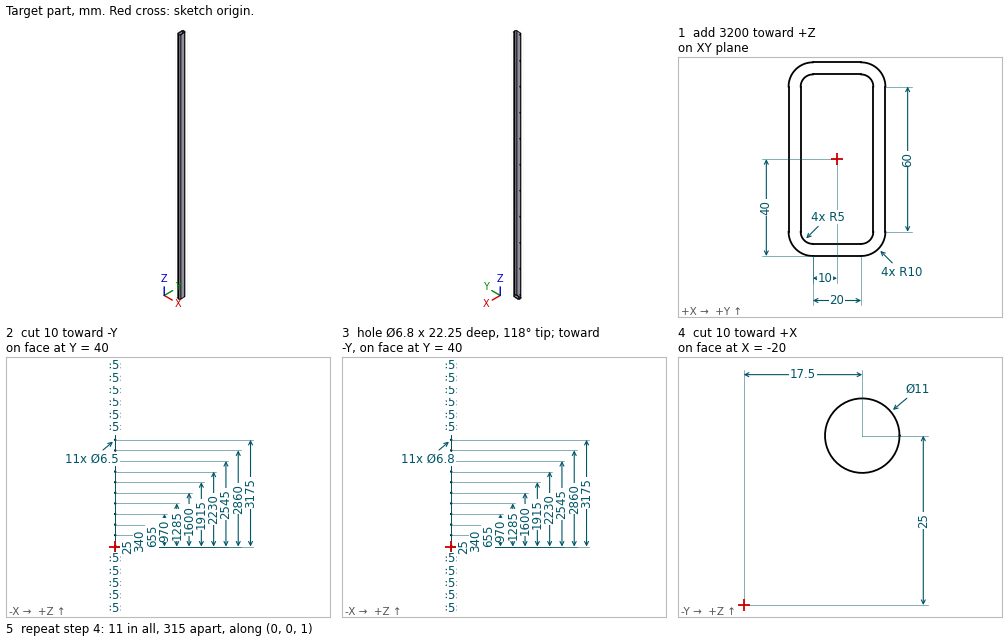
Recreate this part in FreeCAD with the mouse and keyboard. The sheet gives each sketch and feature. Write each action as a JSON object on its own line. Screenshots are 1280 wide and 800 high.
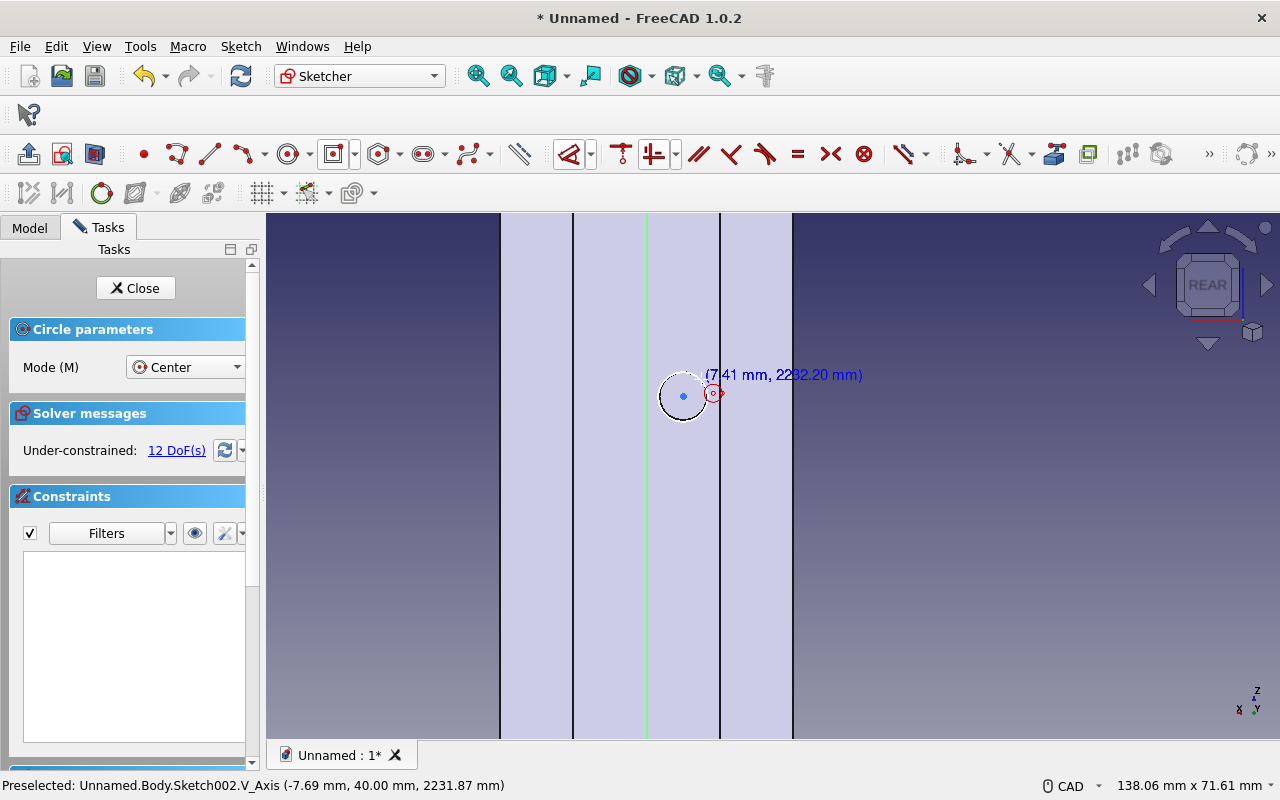
{"action": "scroll", "coordinate": [704, 476], "scroll_direction": "down", "scroll_amount": 15}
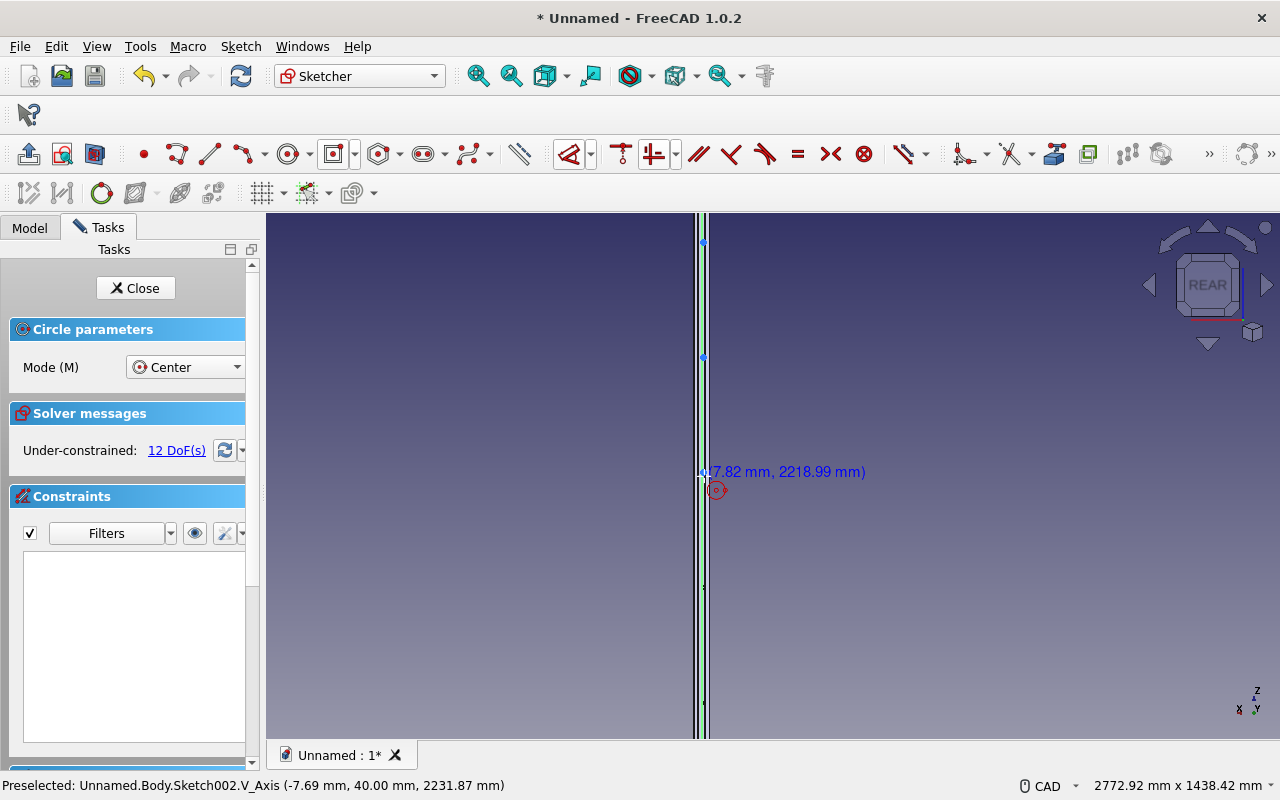
{"action": "scroll", "coordinate": [705, 377], "scroll_direction": "down", "scroll_amount": 6}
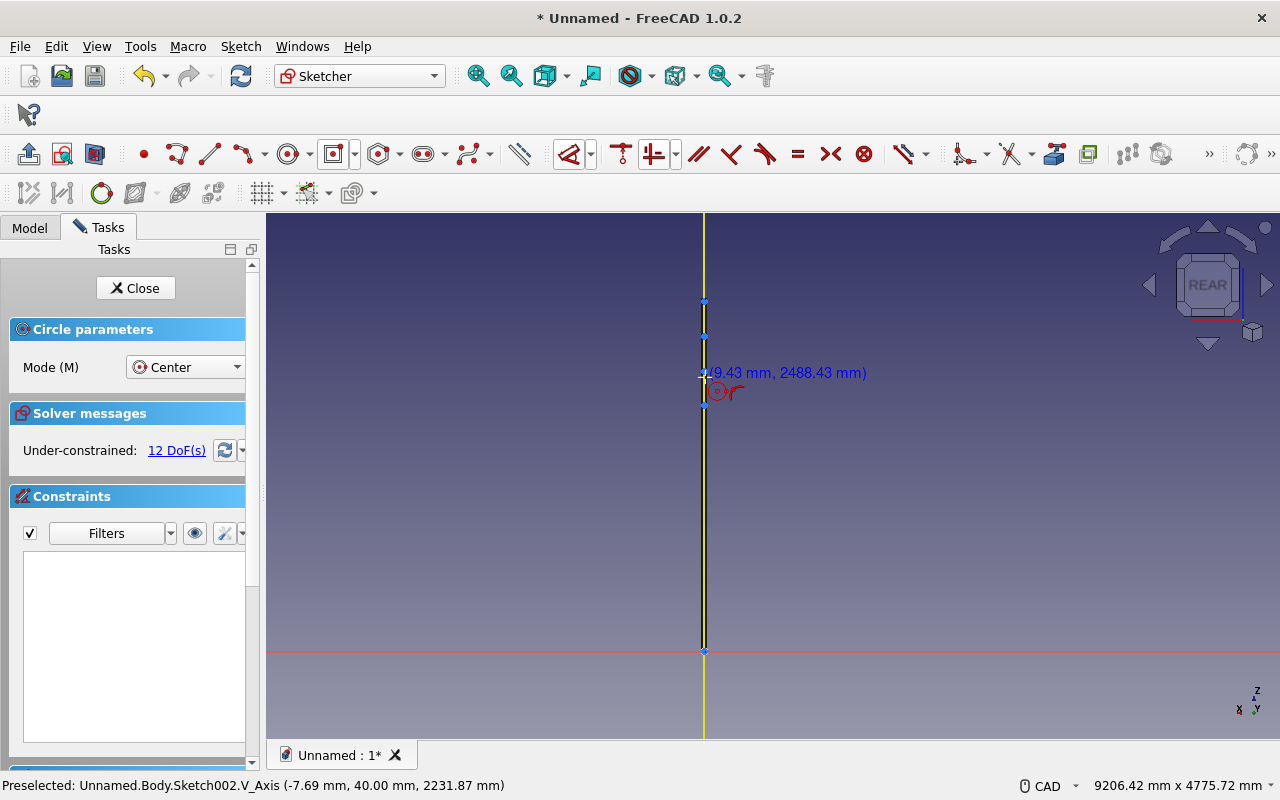
{"action": "scroll", "coordinate": [705, 441], "scroll_direction": "up", "scroll_amount": 21}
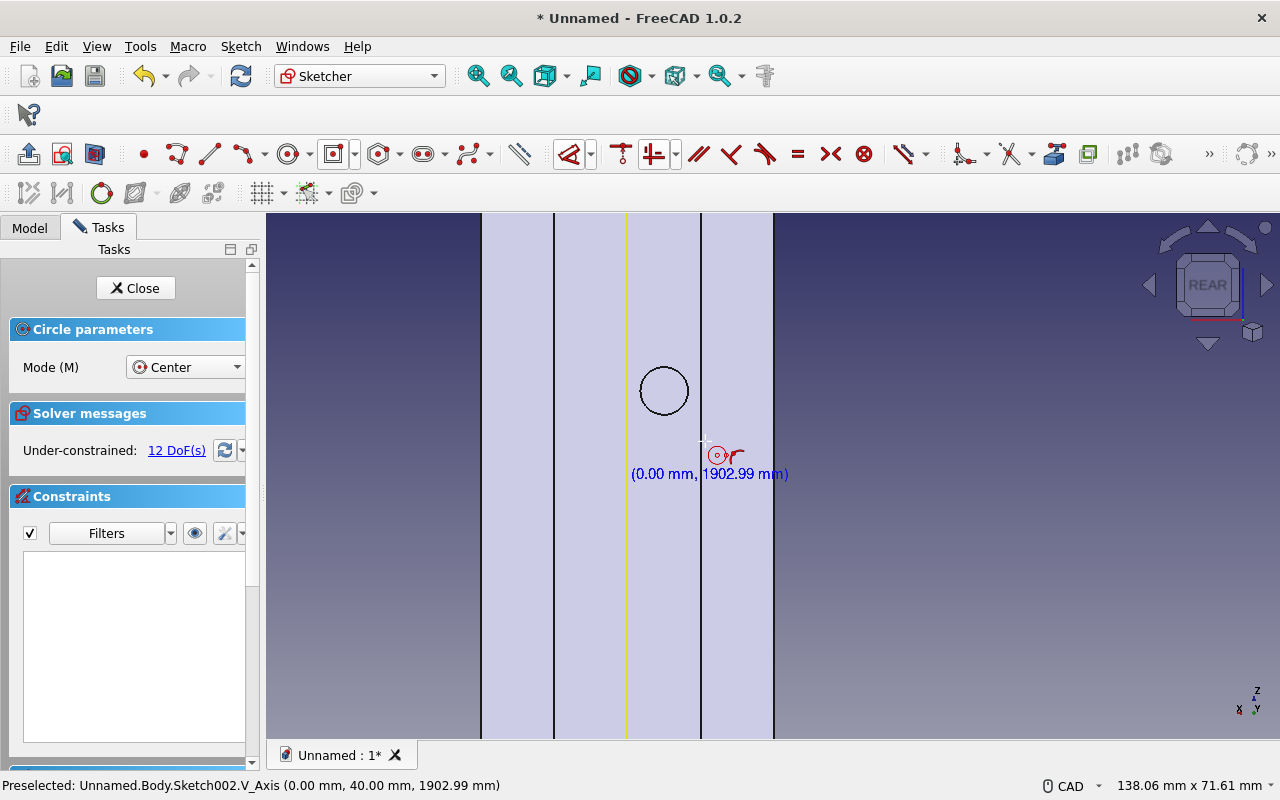
{"action": "left_click", "coordinate": [664, 391]}
{"action": "left_click", "coordinate": [682, 373]}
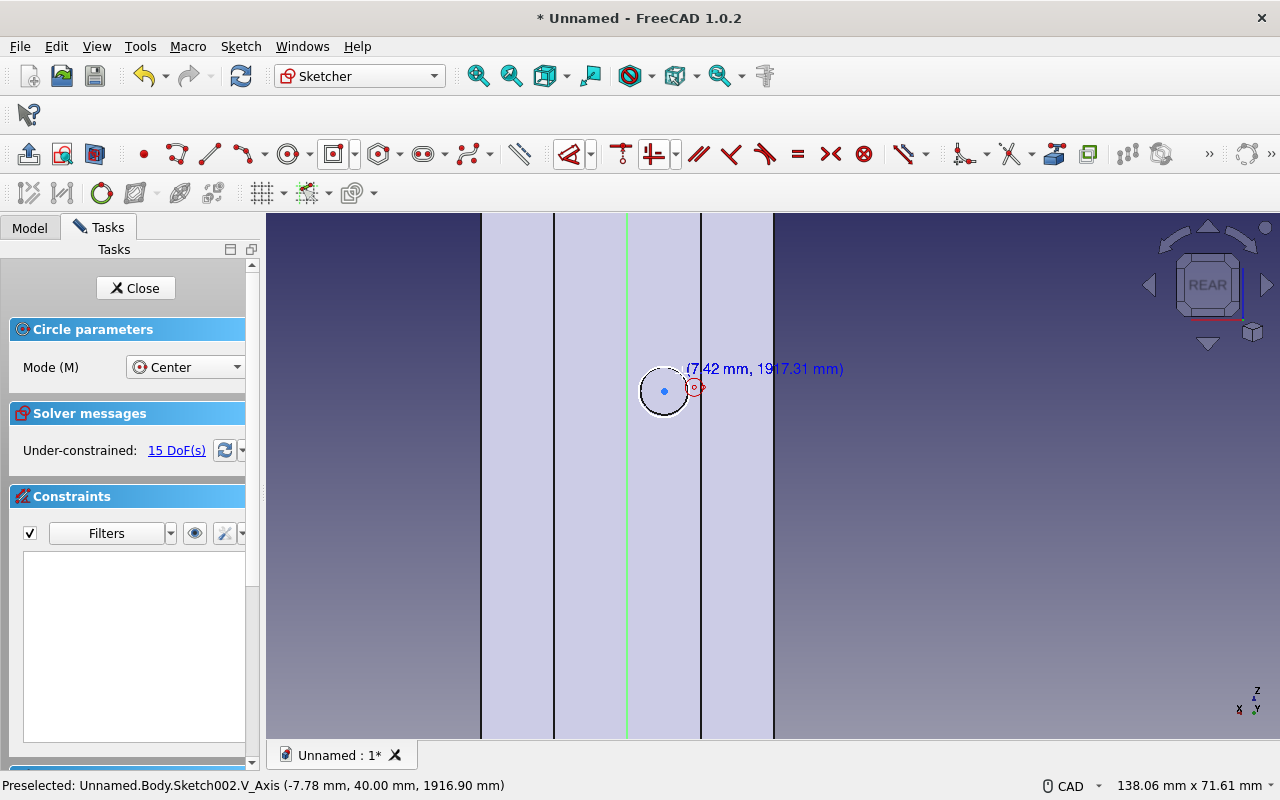
{"action": "scroll", "coordinate": [704, 476], "scroll_direction": "down", "scroll_amount": 15}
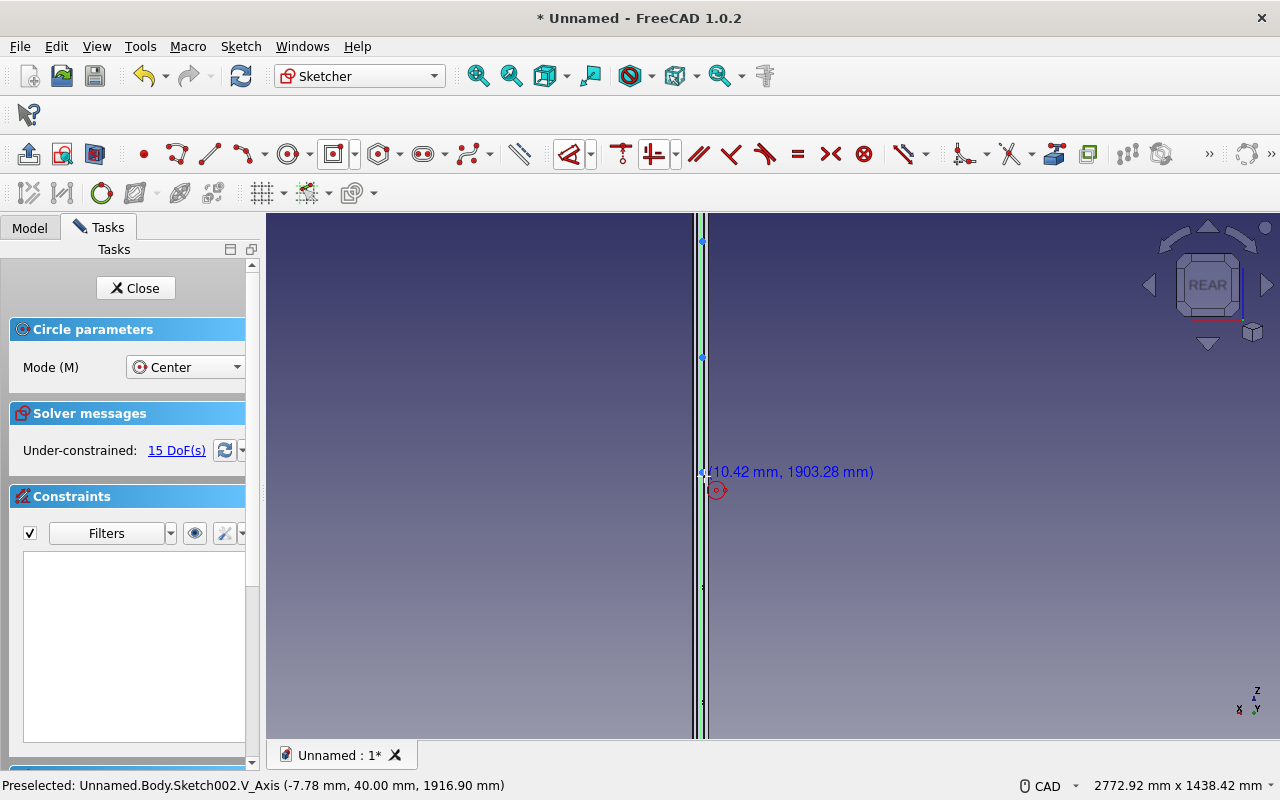
{"action": "scroll", "coordinate": [706, 426], "scroll_direction": "down", "scroll_amount": 6}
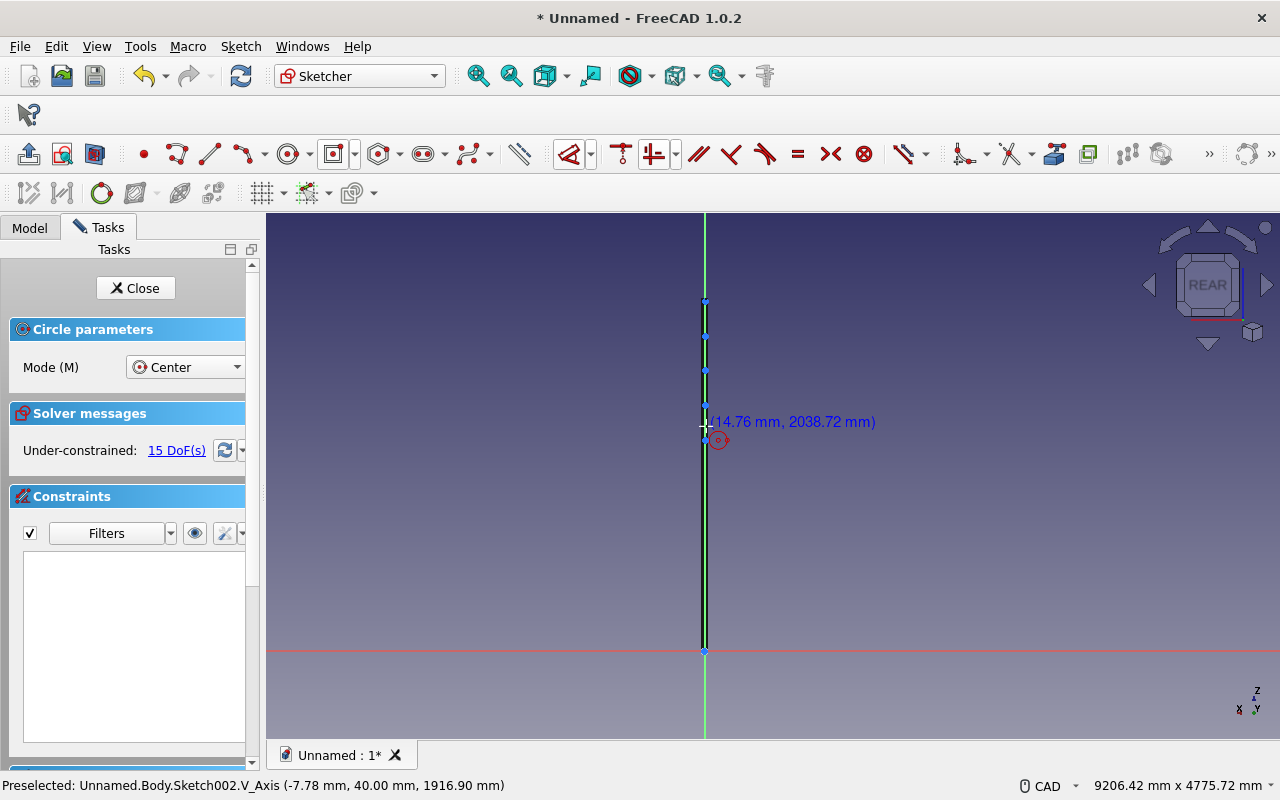
{"action": "scroll", "coordinate": [705, 475], "scroll_direction": "up", "scroll_amount": 21}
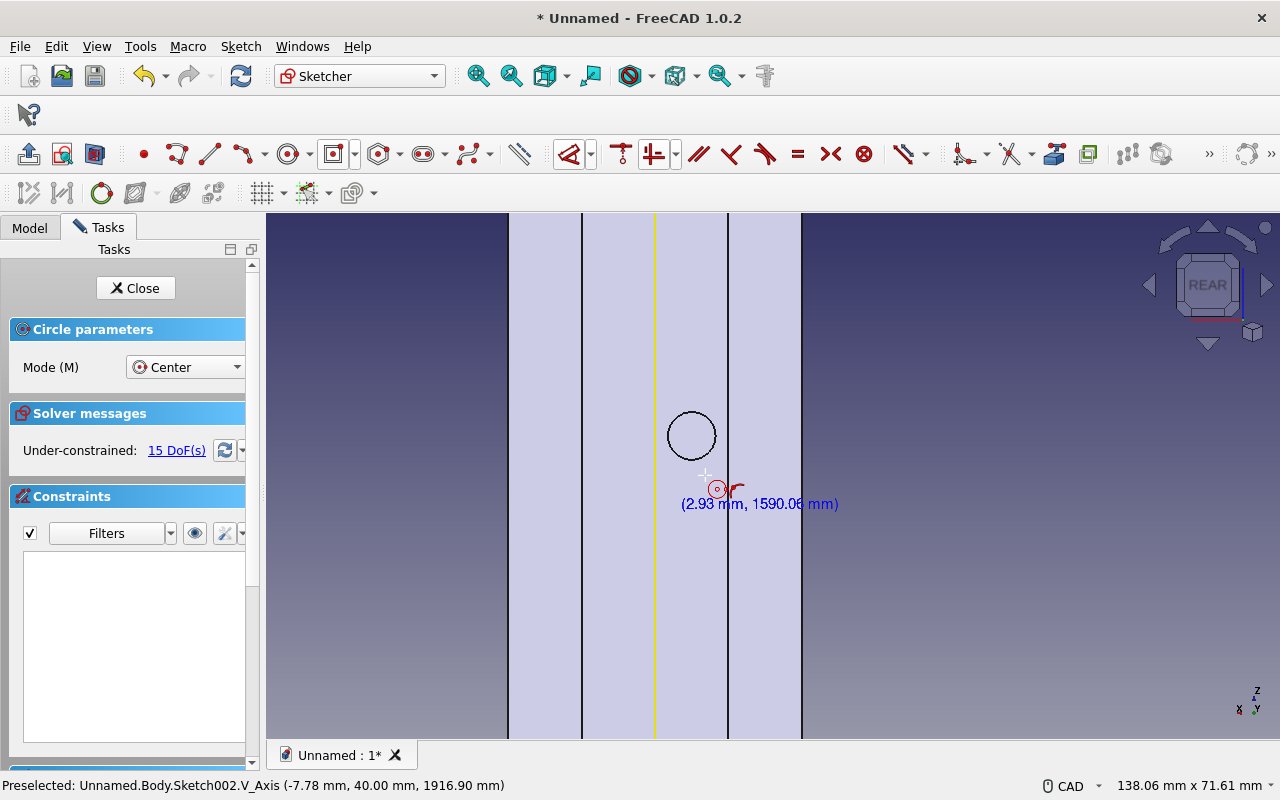
{"action": "left_click", "coordinate": [692, 436]}
{"action": "left_click", "coordinate": [709, 418]}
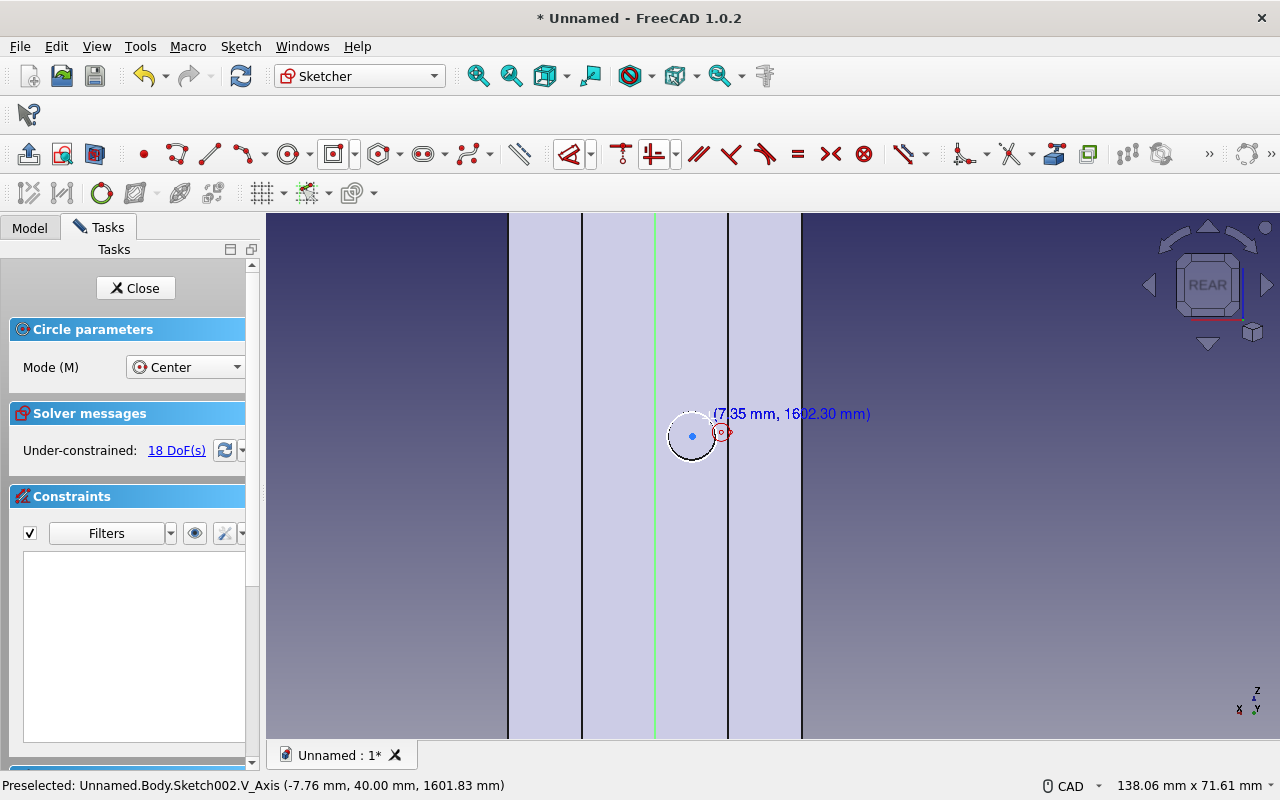
{"action": "scroll", "coordinate": [704, 476], "scroll_direction": "down", "scroll_amount": 15}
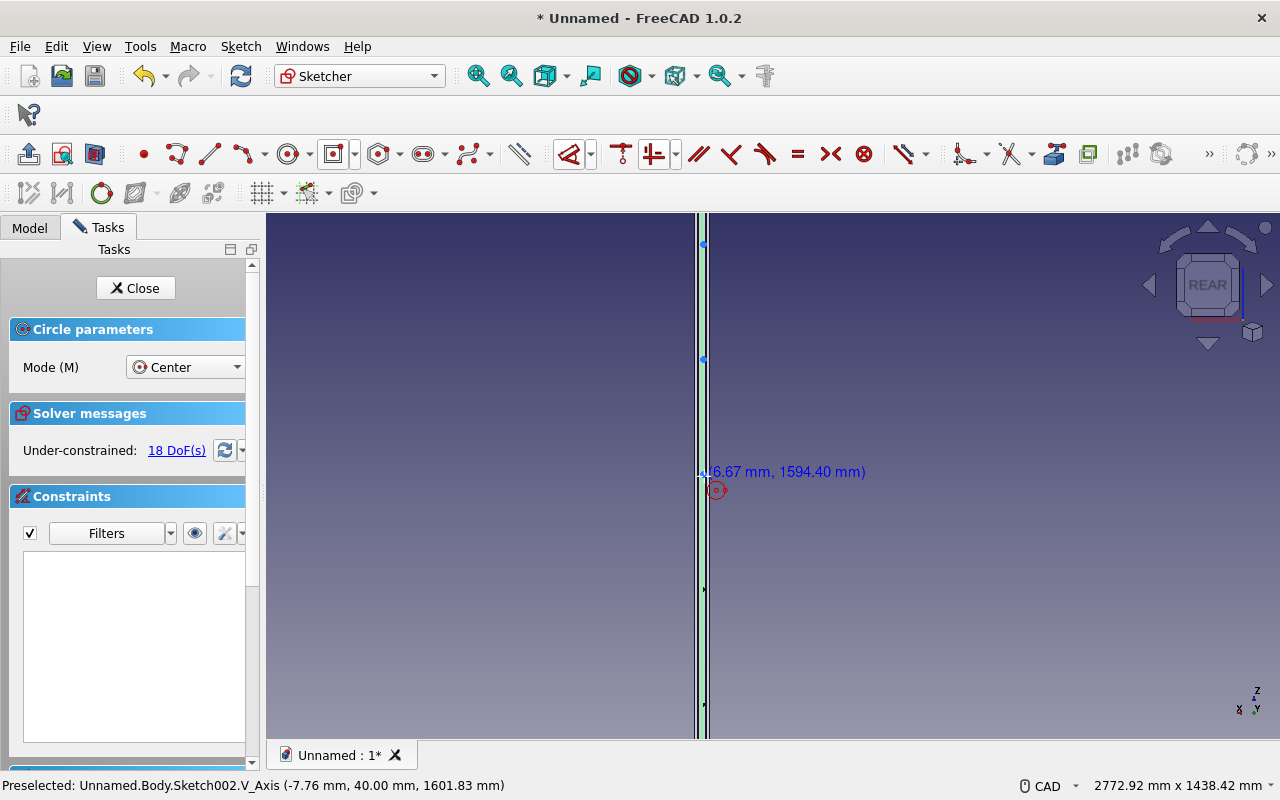
{"action": "scroll", "coordinate": [705, 475], "scroll_direction": "down", "scroll_amount": 6}